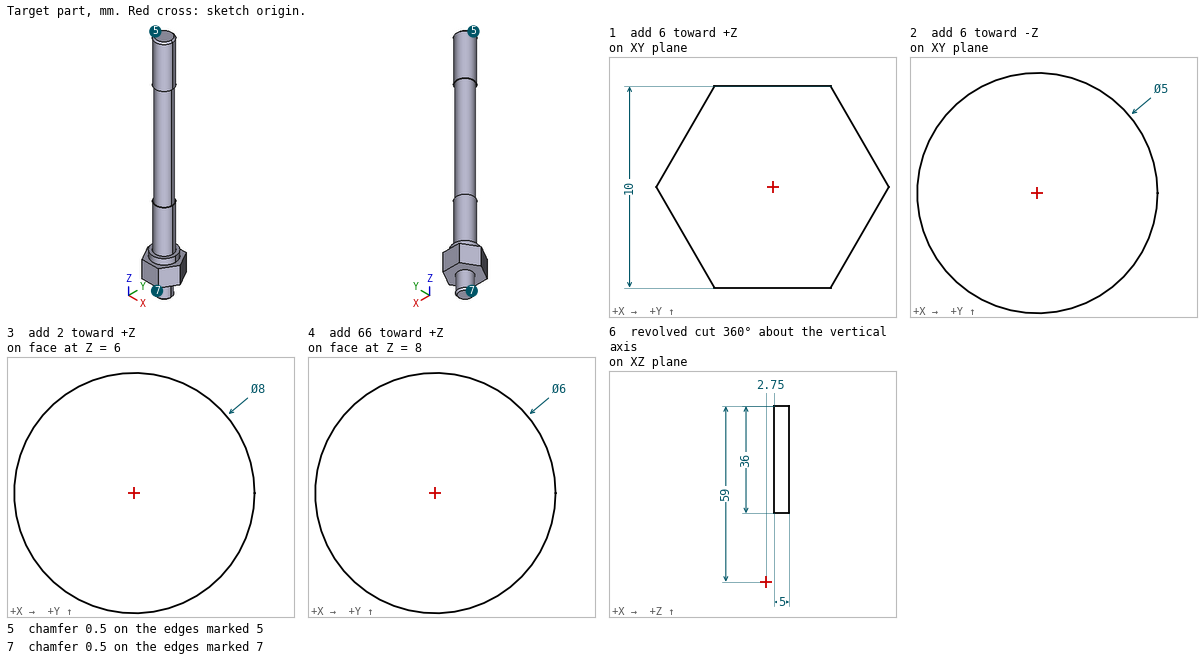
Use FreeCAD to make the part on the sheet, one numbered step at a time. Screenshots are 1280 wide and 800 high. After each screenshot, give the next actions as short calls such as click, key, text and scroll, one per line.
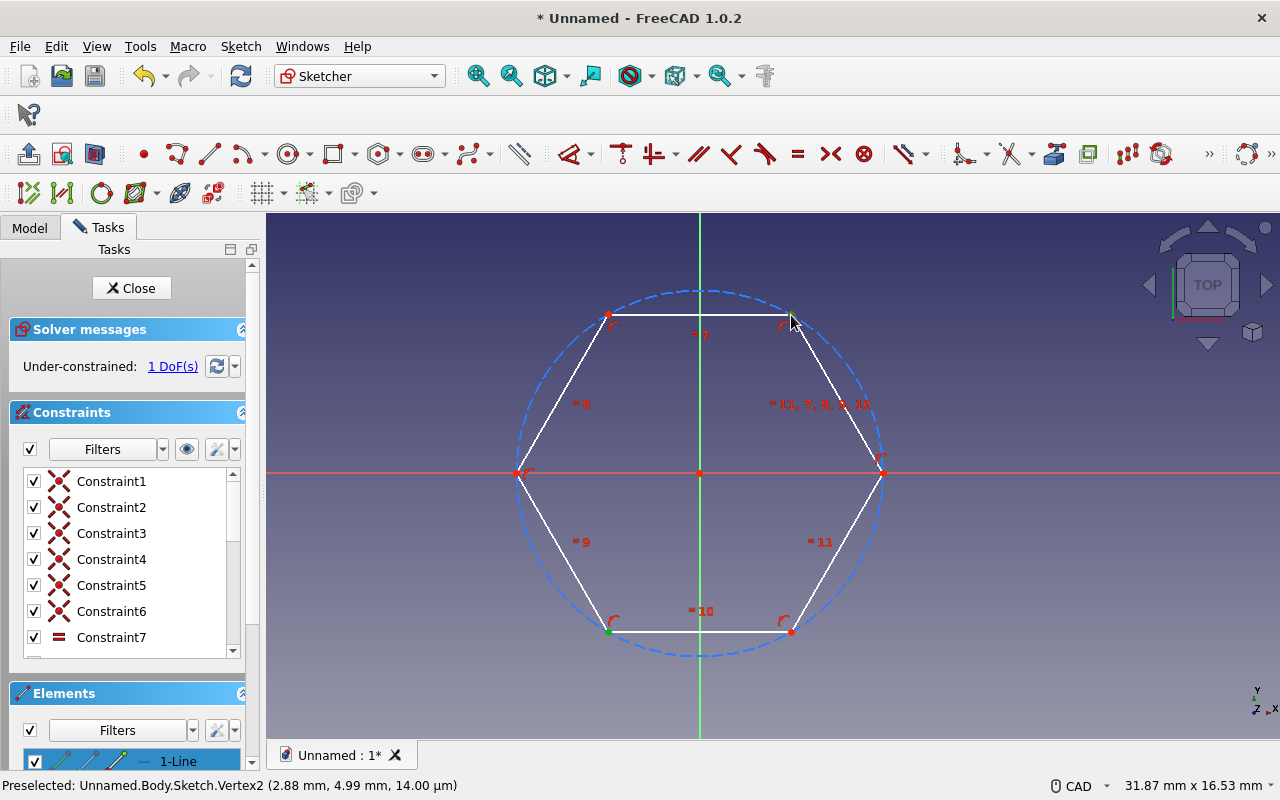
click(590, 154)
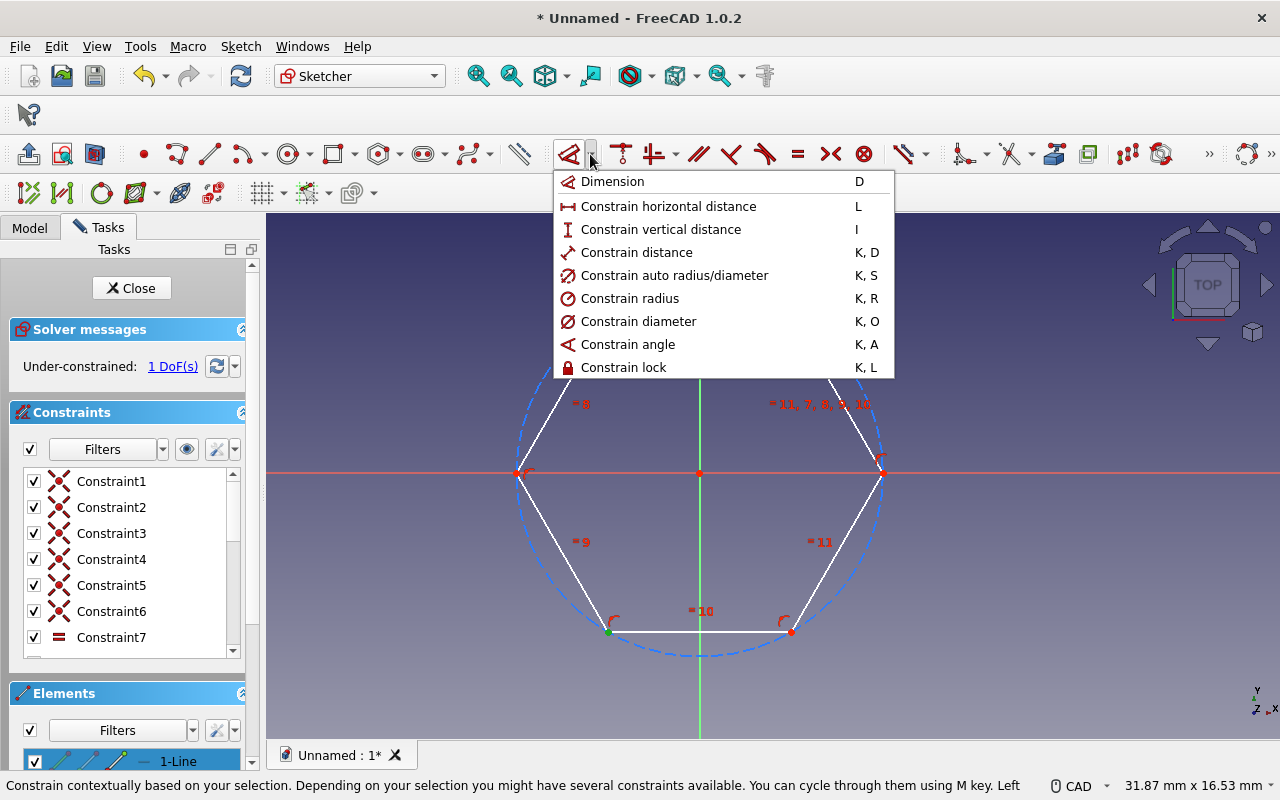
click(724, 230)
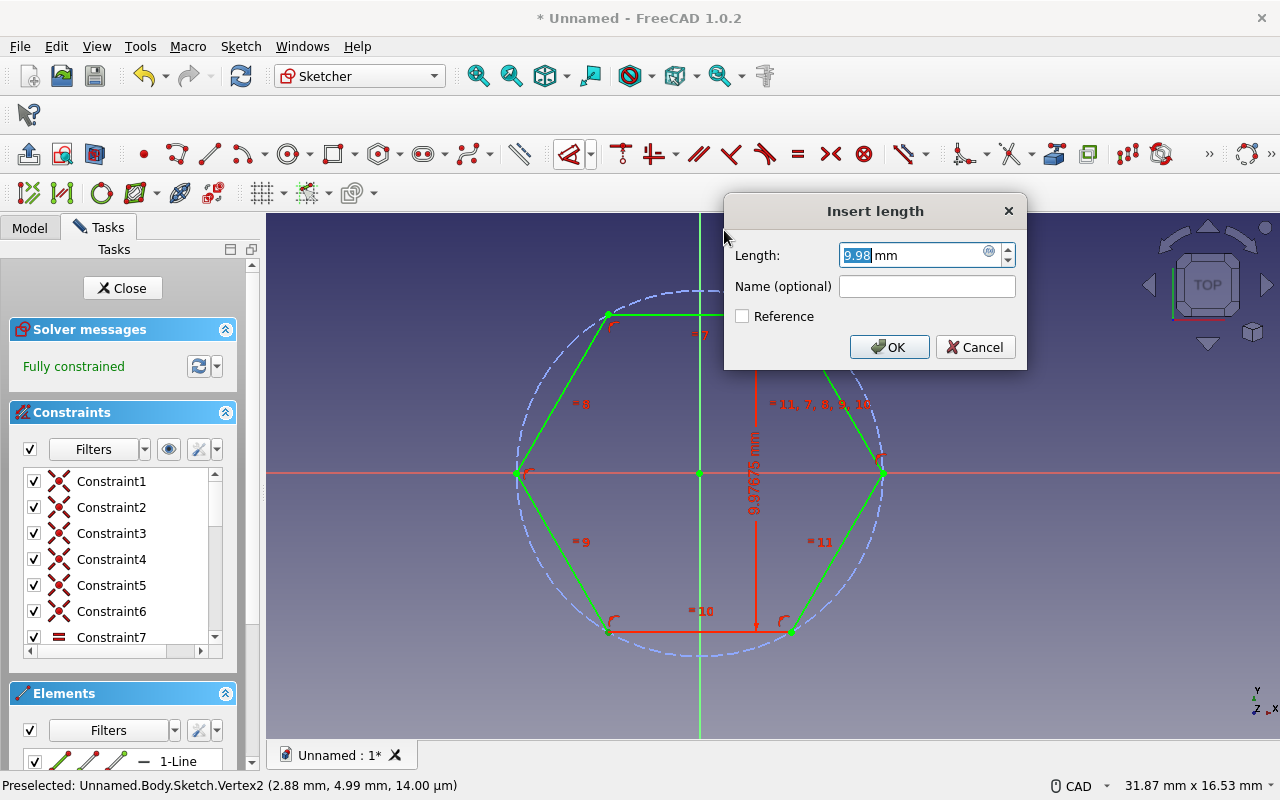
text(10)
key(Return)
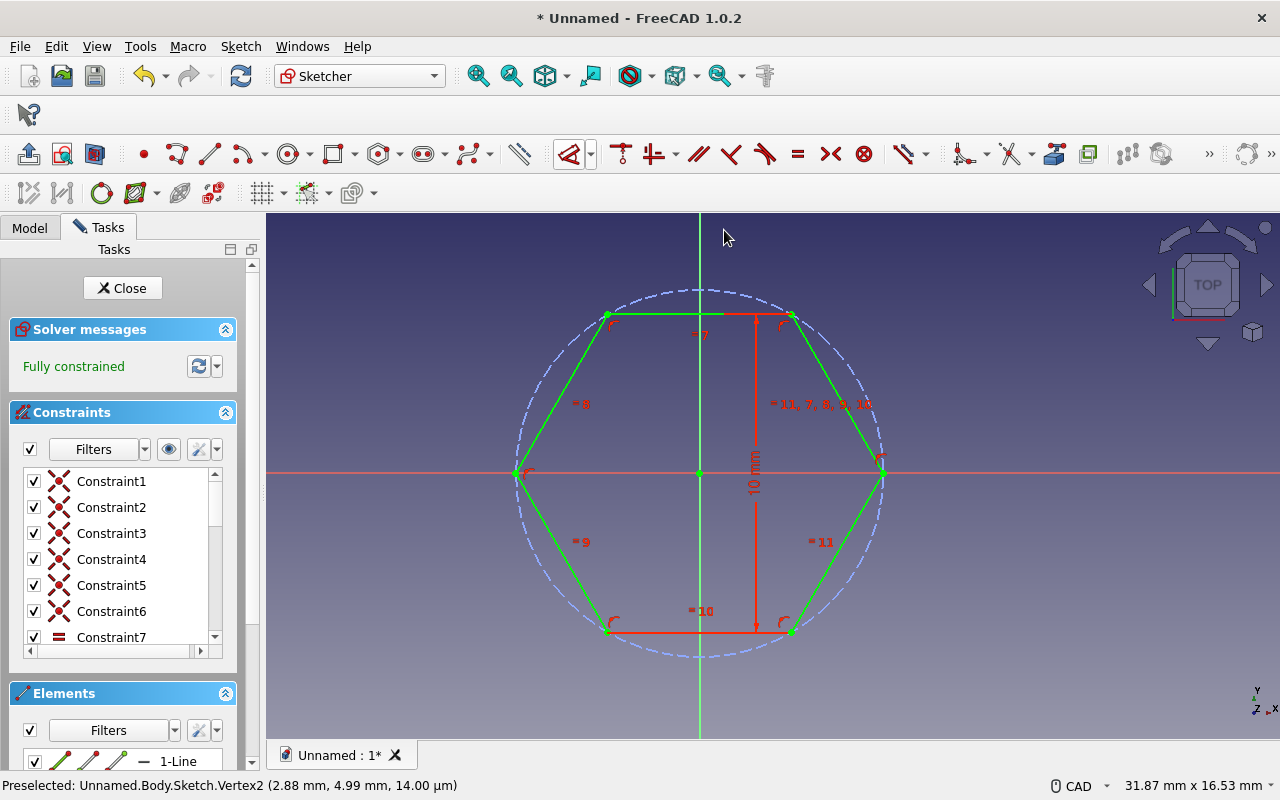
click(123, 288)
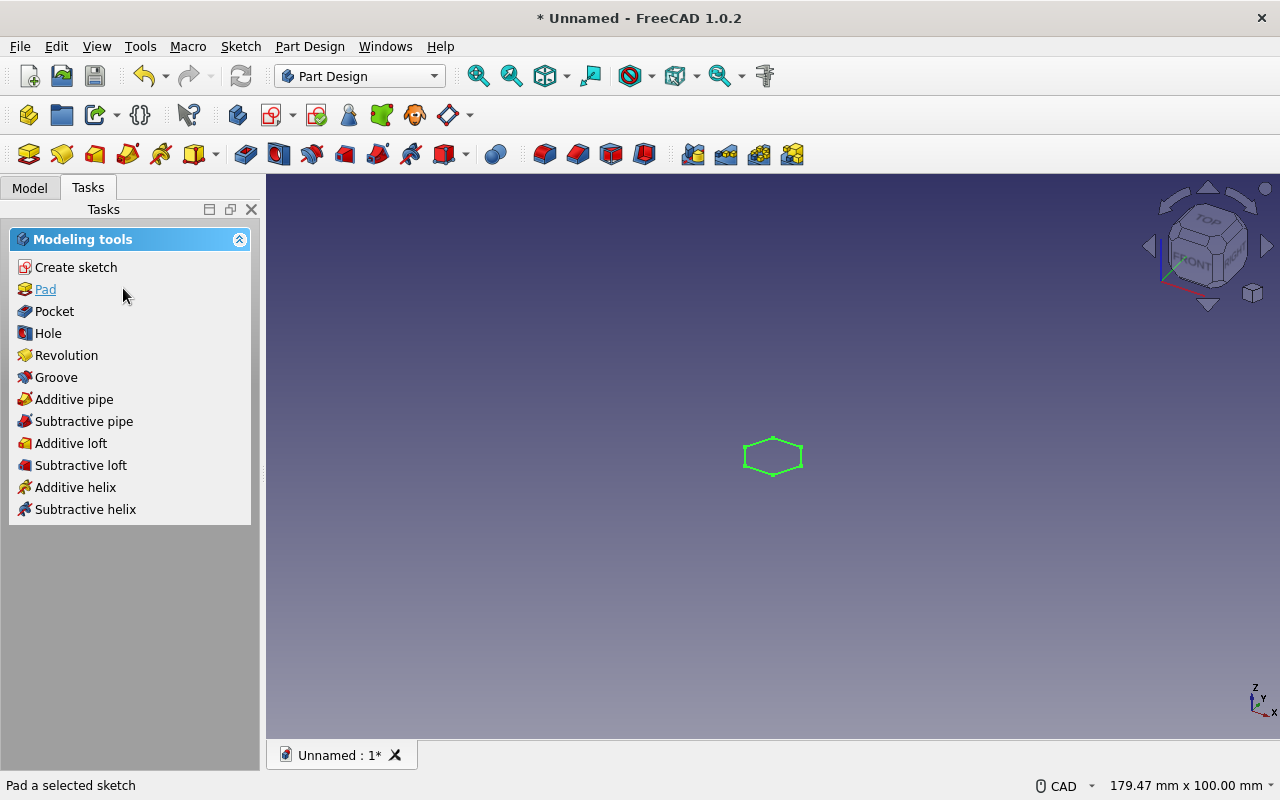
click(29, 154)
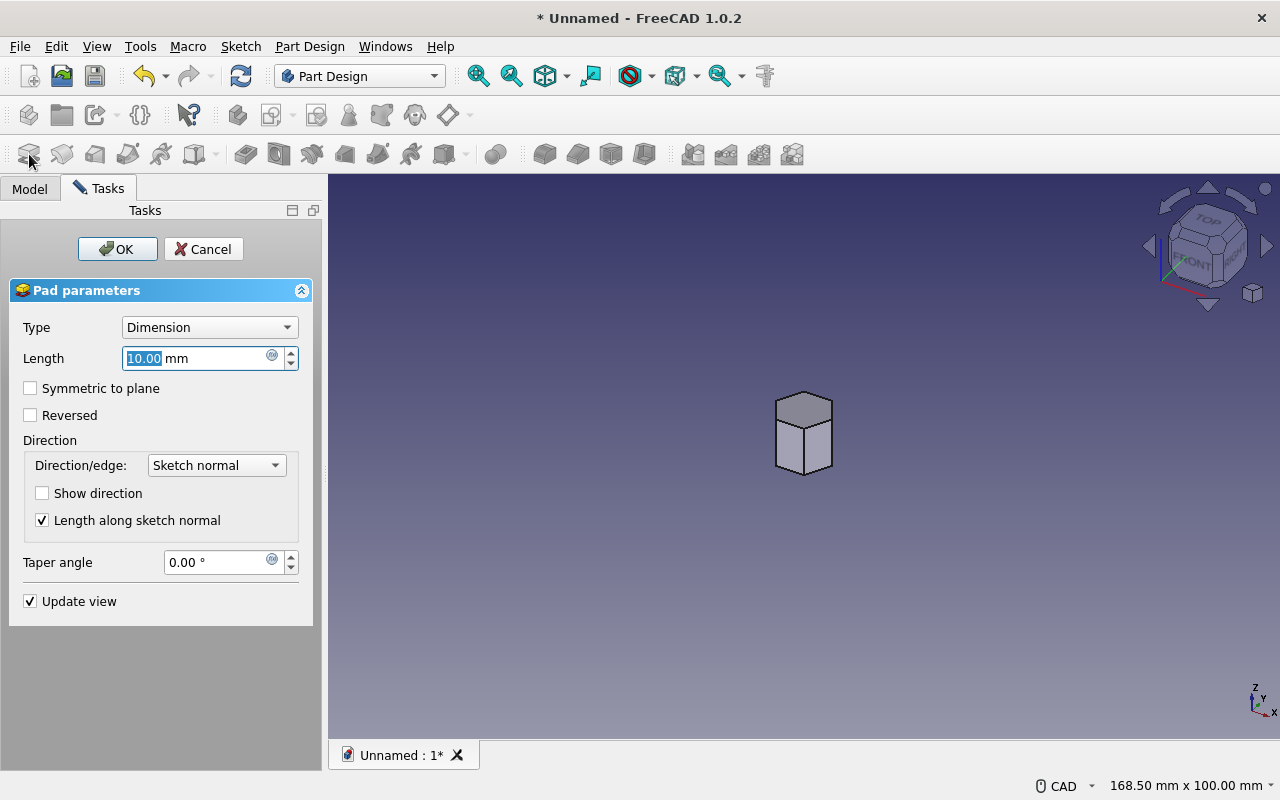
text(6)
key(Tab)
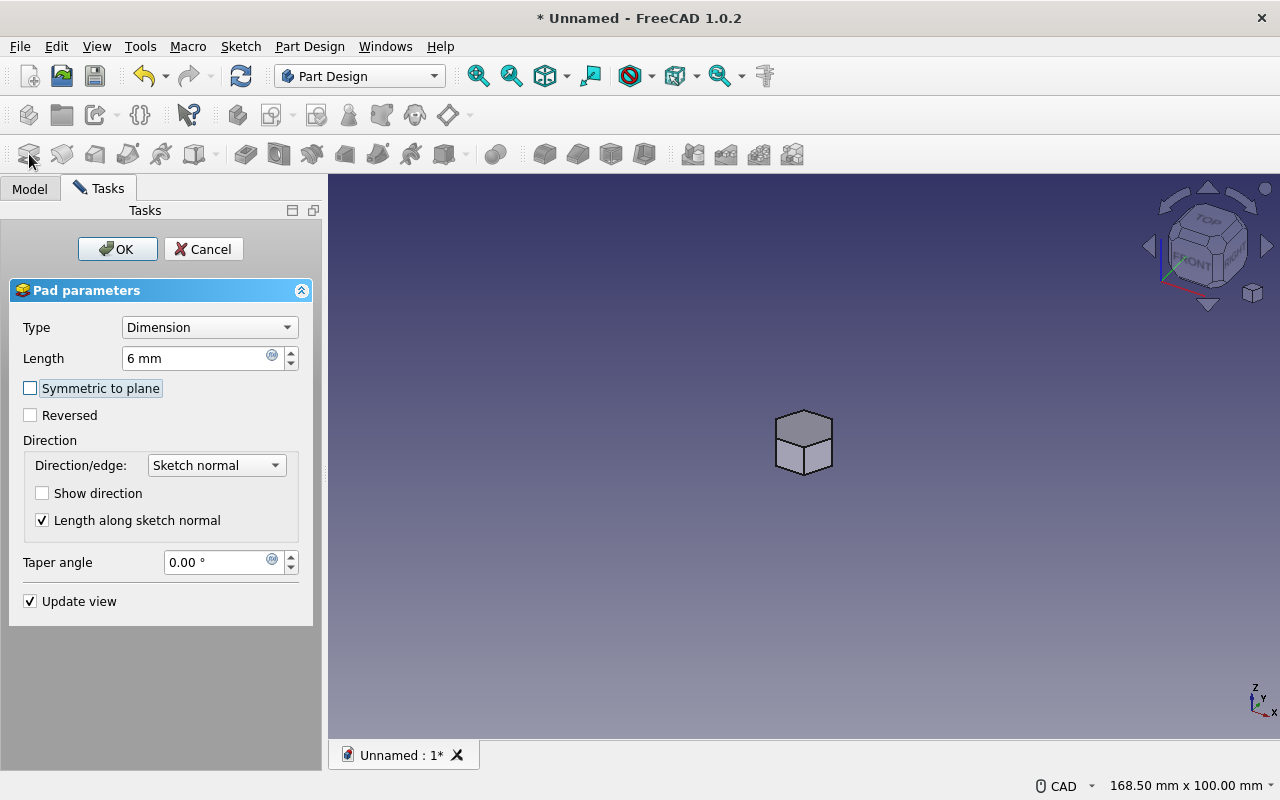
click(118, 249)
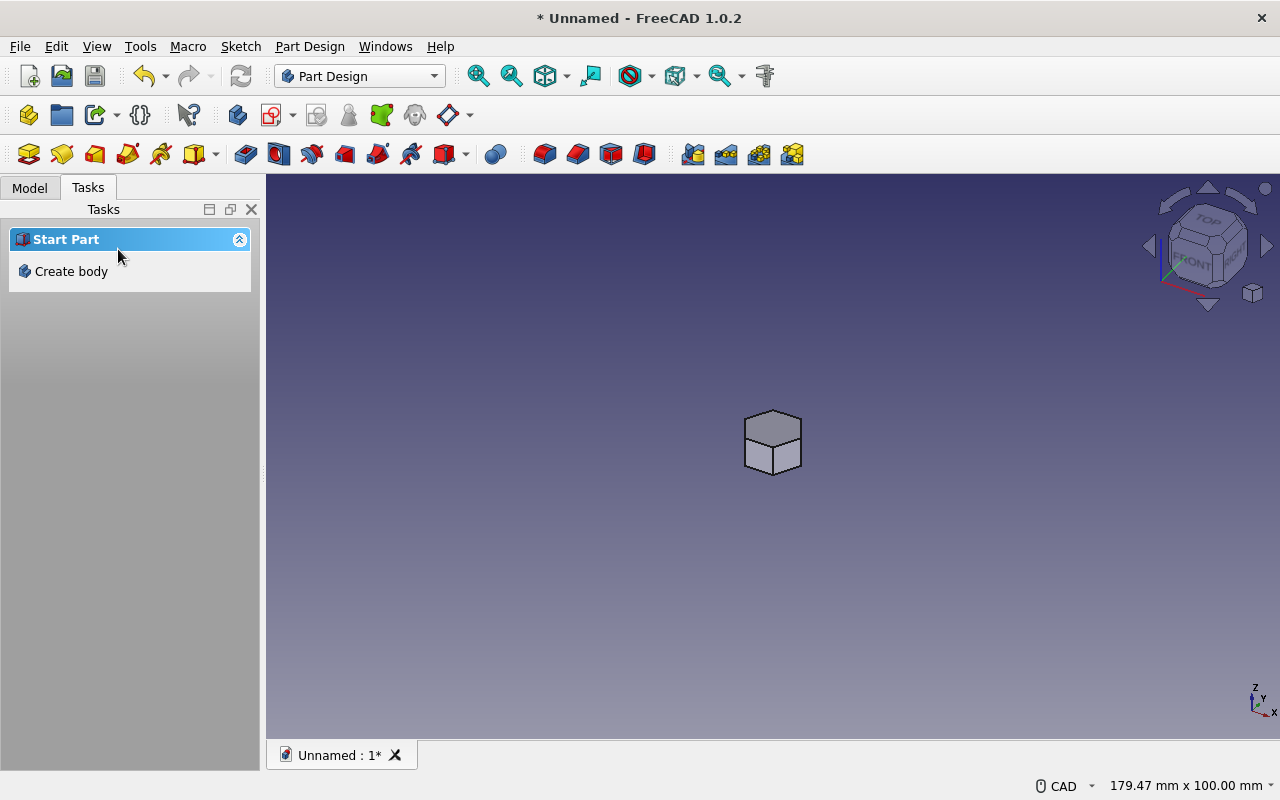
click(479, 76)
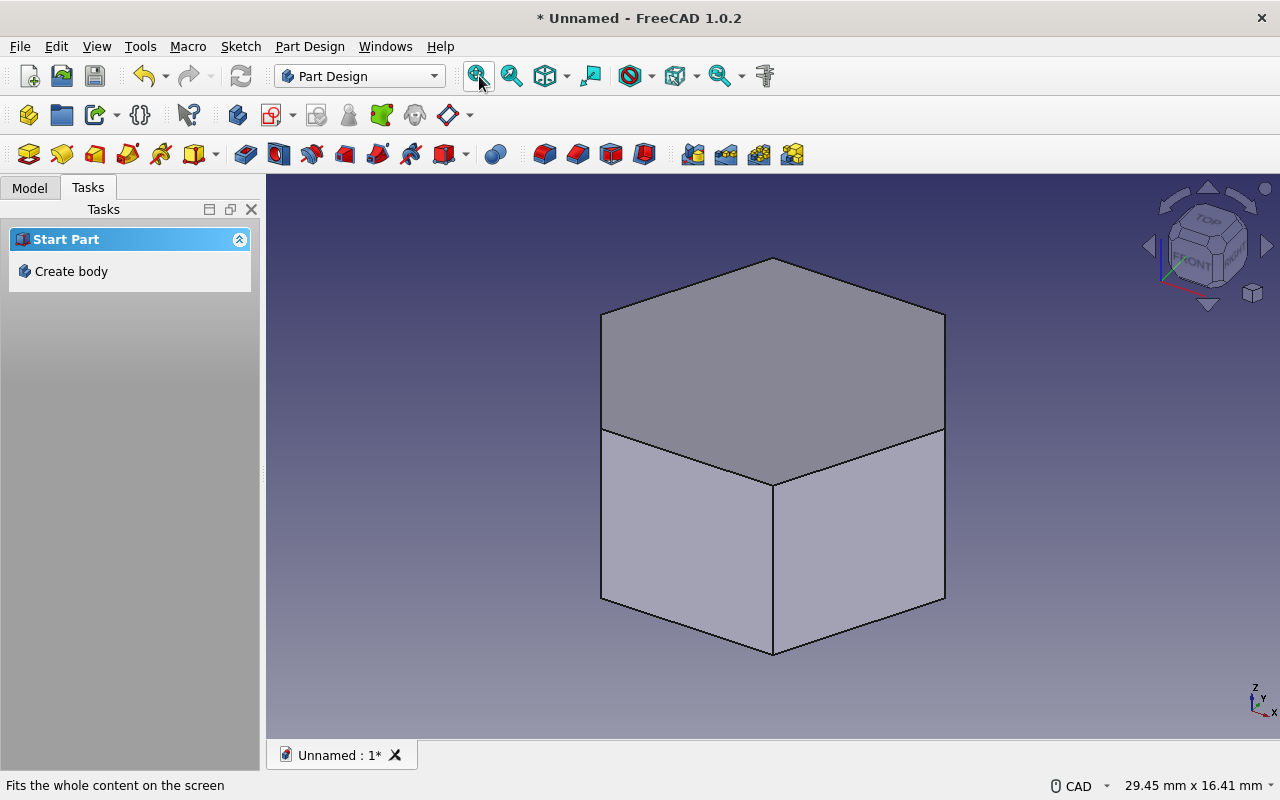
click(270, 116)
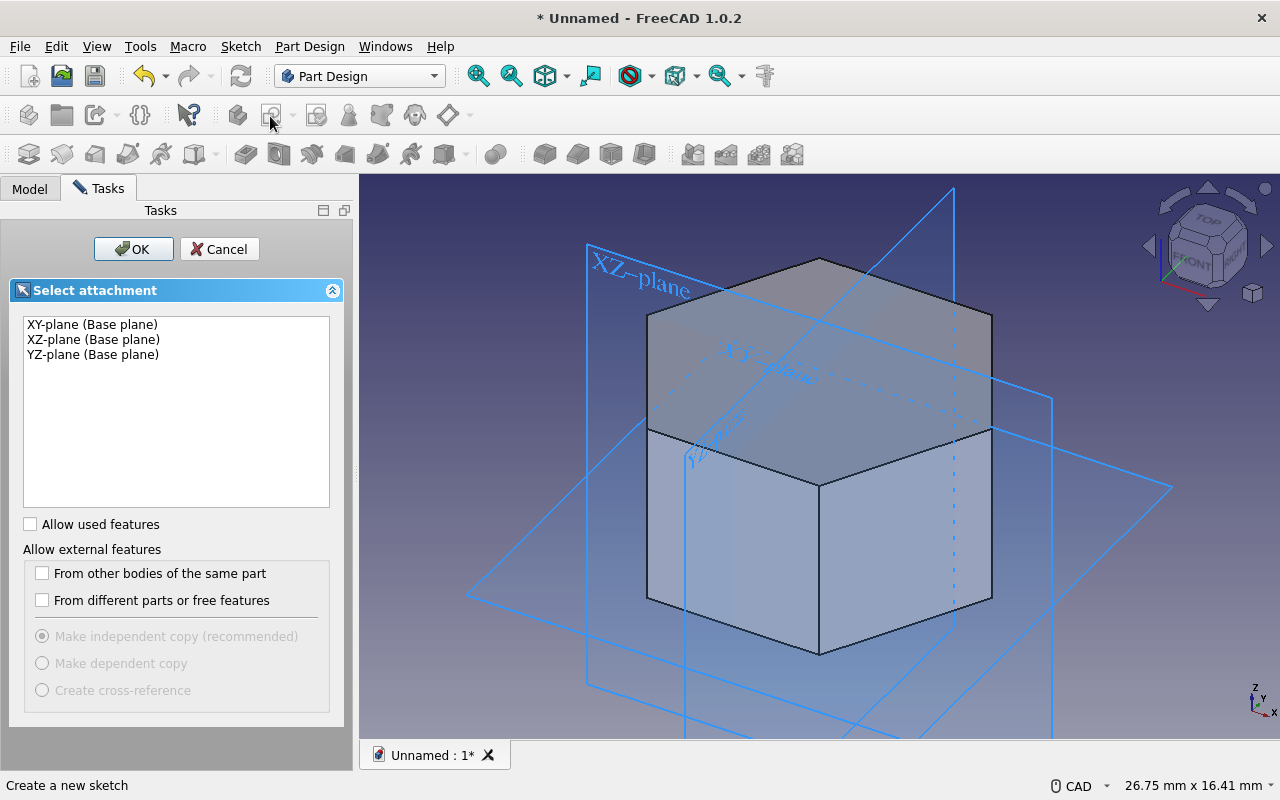
click(84, 324)